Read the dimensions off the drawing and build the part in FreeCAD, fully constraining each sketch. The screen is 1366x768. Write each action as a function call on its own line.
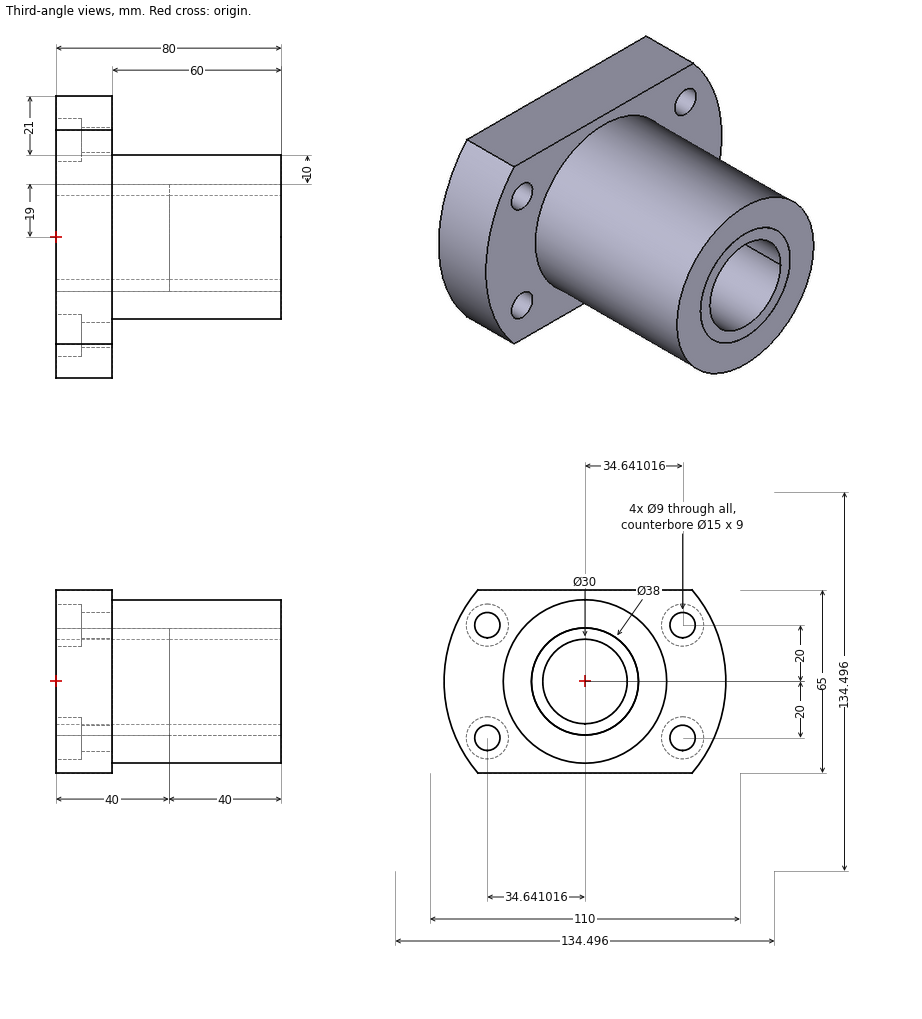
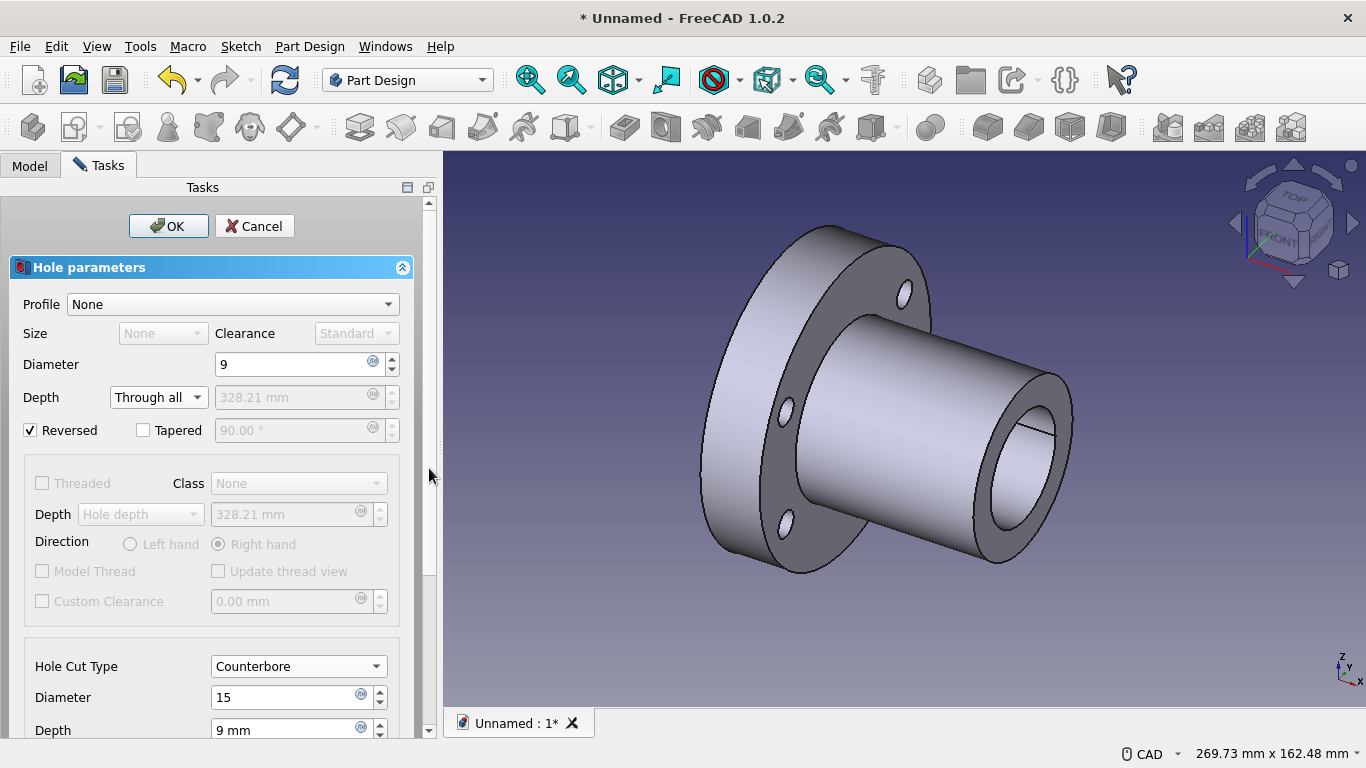
click(169, 226)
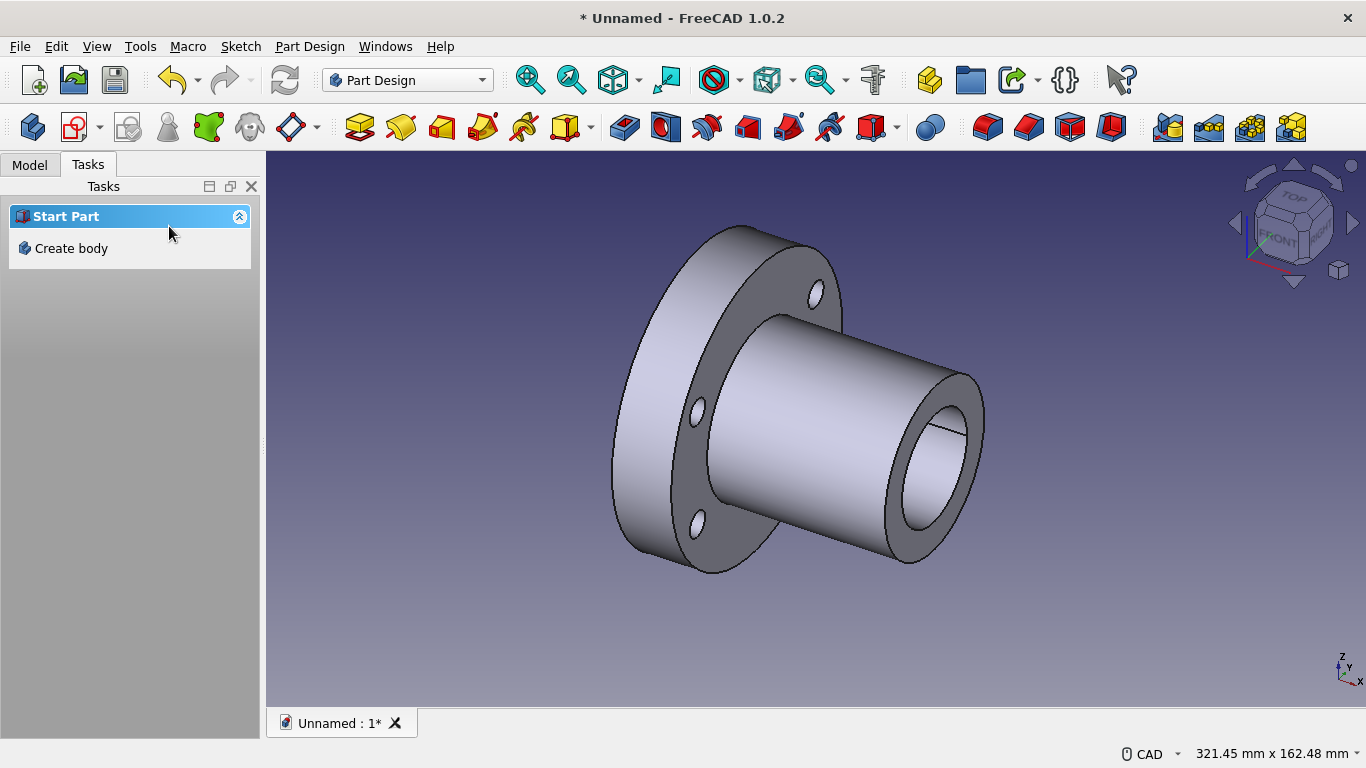
click(74, 128)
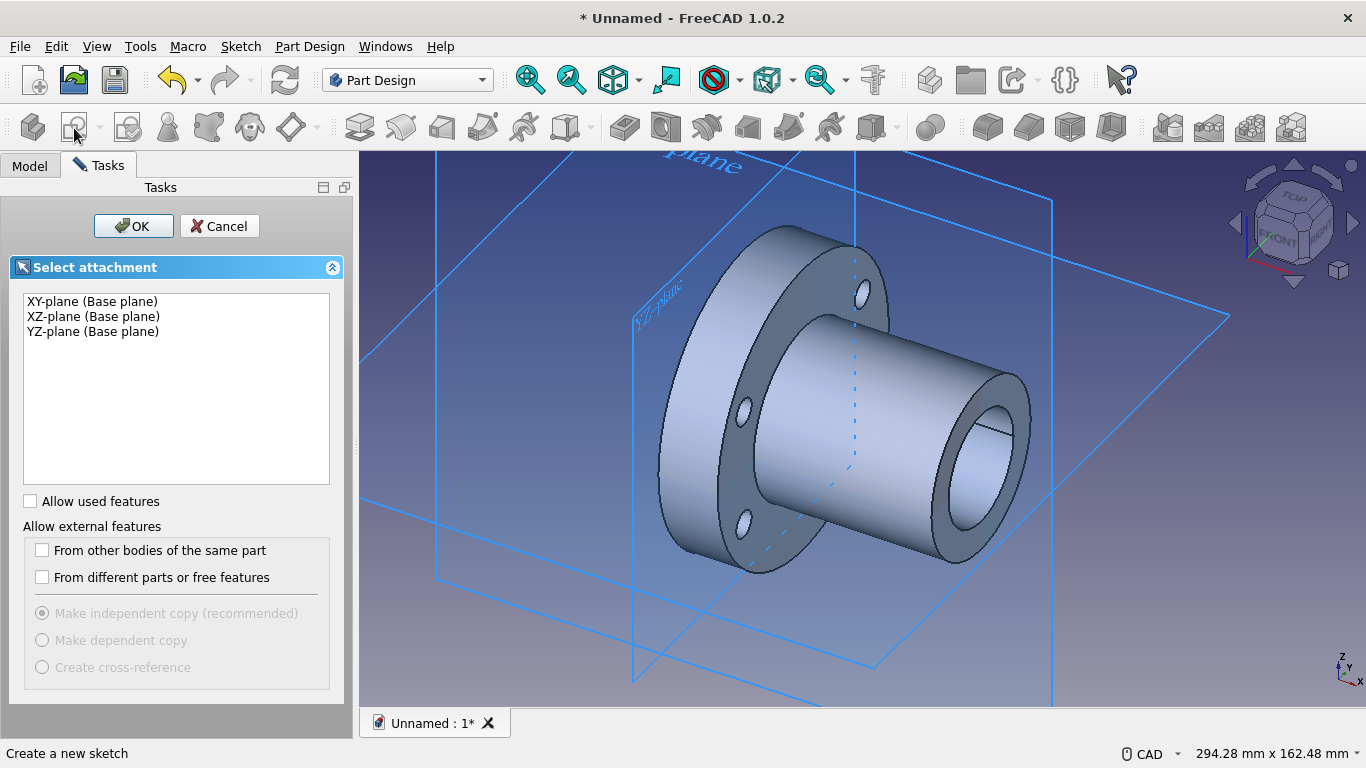
click(84, 332)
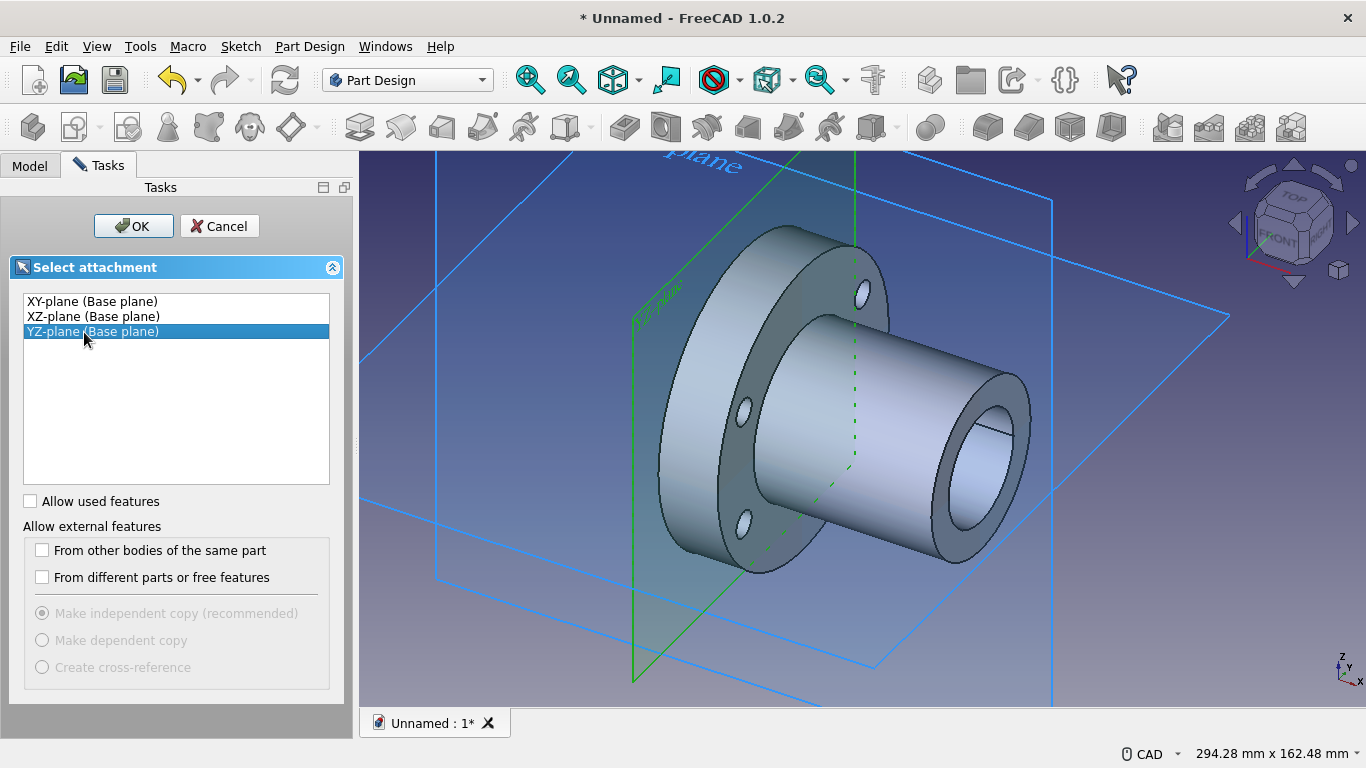
click(134, 226)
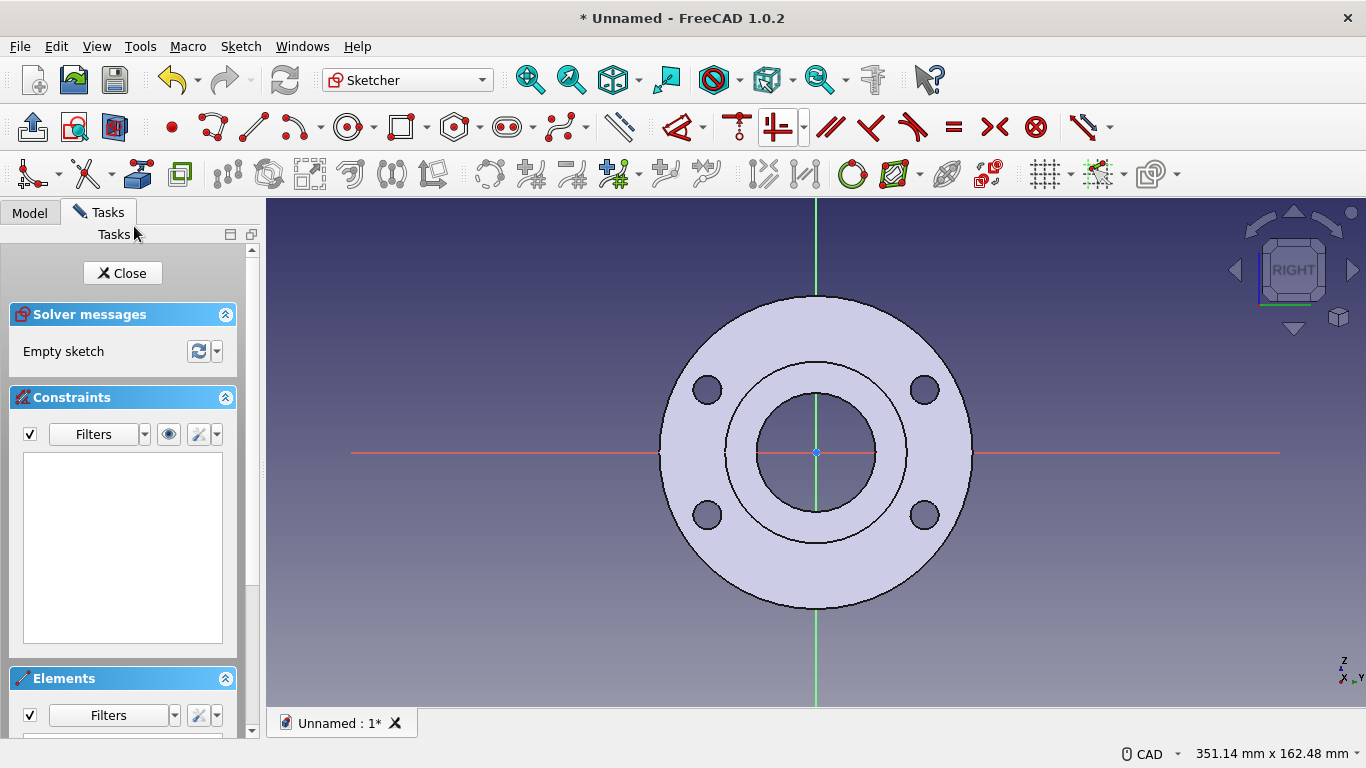
click(115, 128)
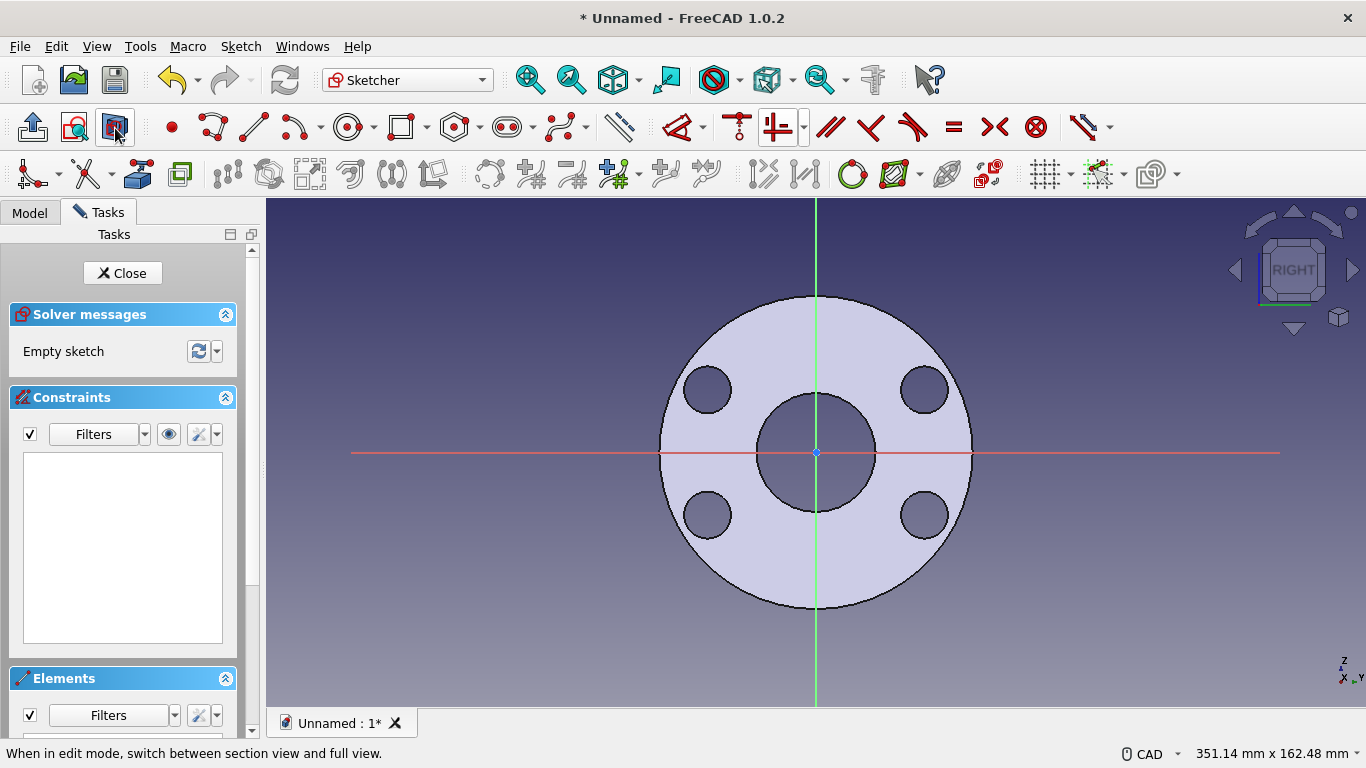
scroll(438, 452, down, 1)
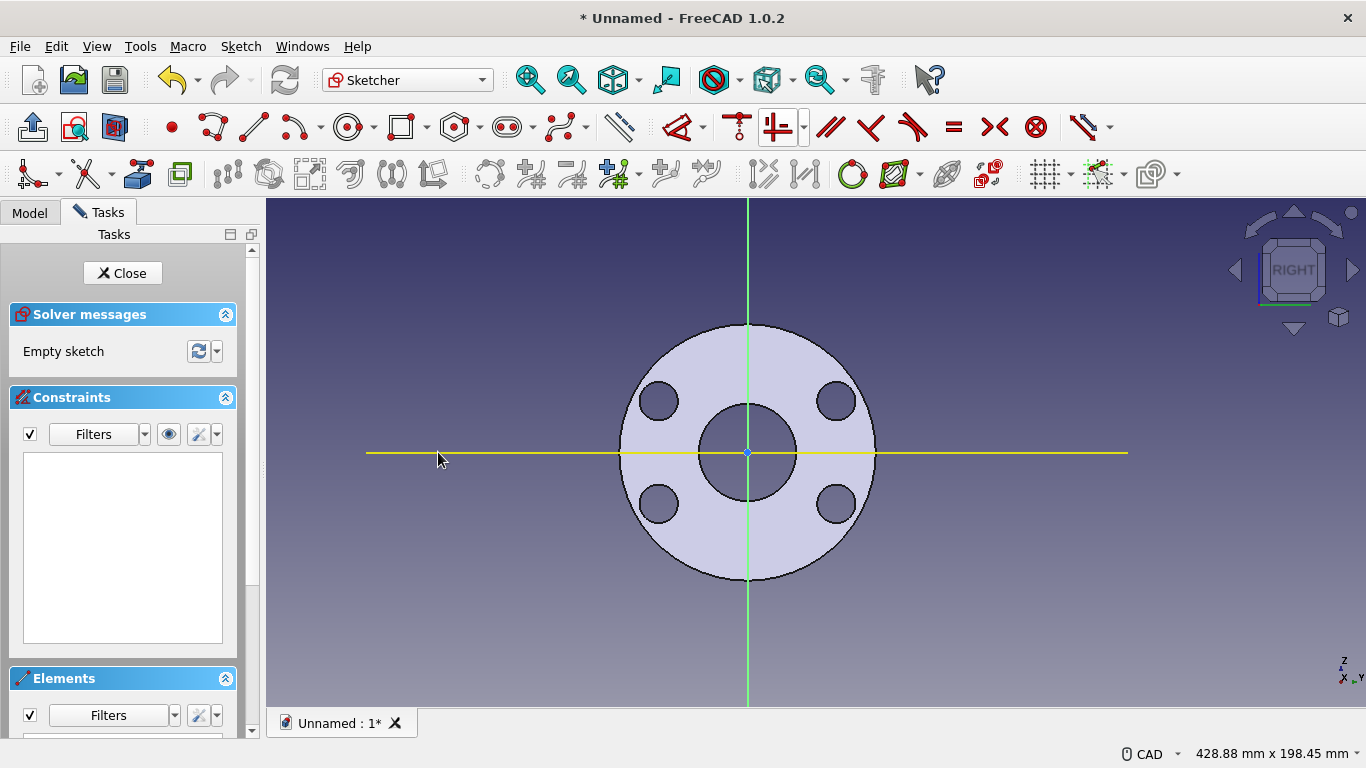
key(g)
key(v)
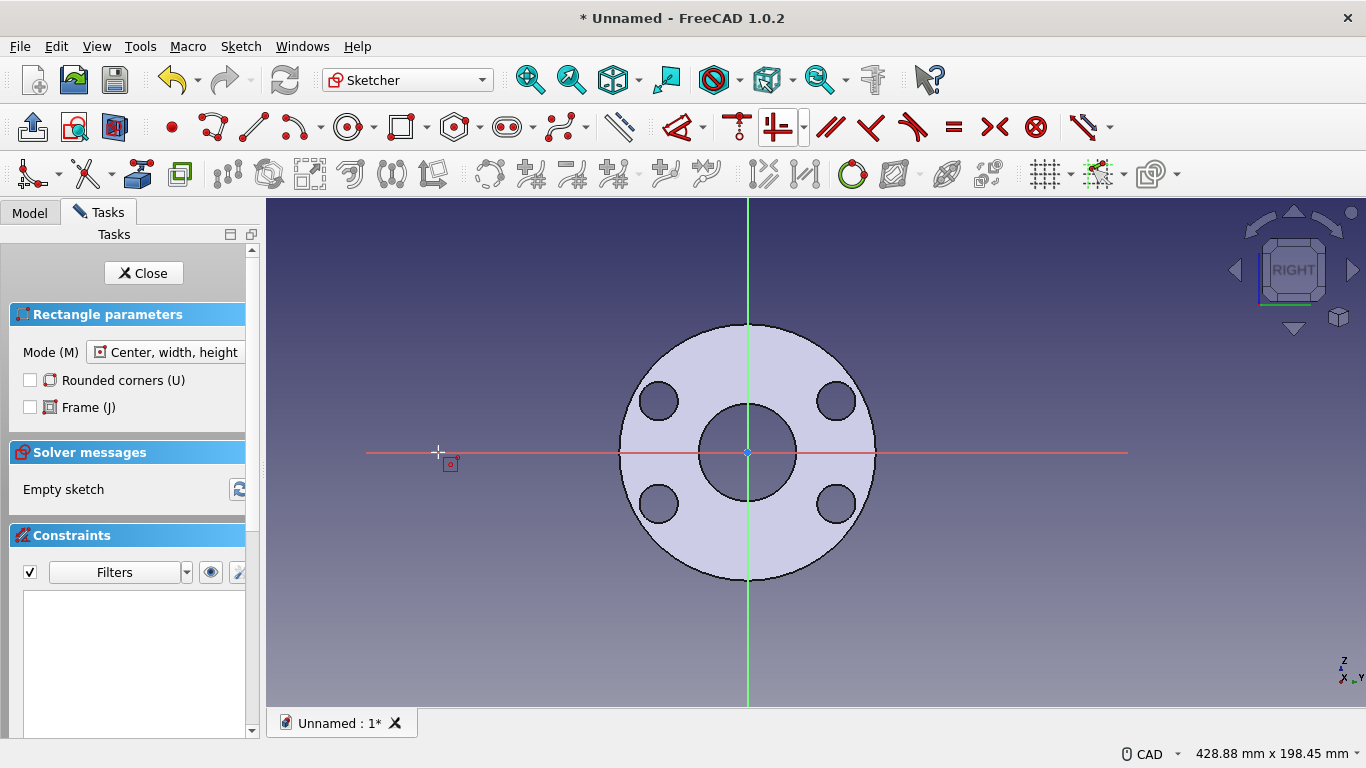
click(748, 452)
click(920, 280)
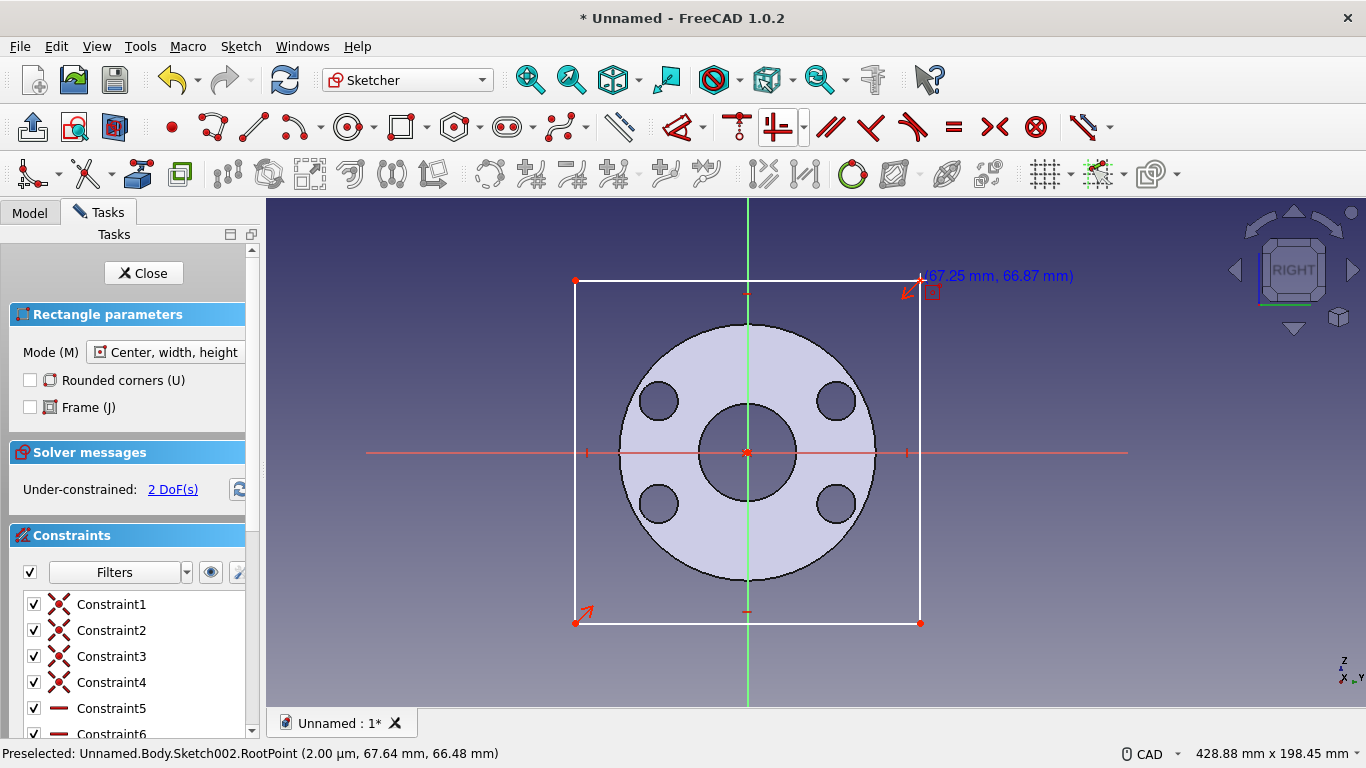
click(748, 452)
click(889, 369)
key(Escape)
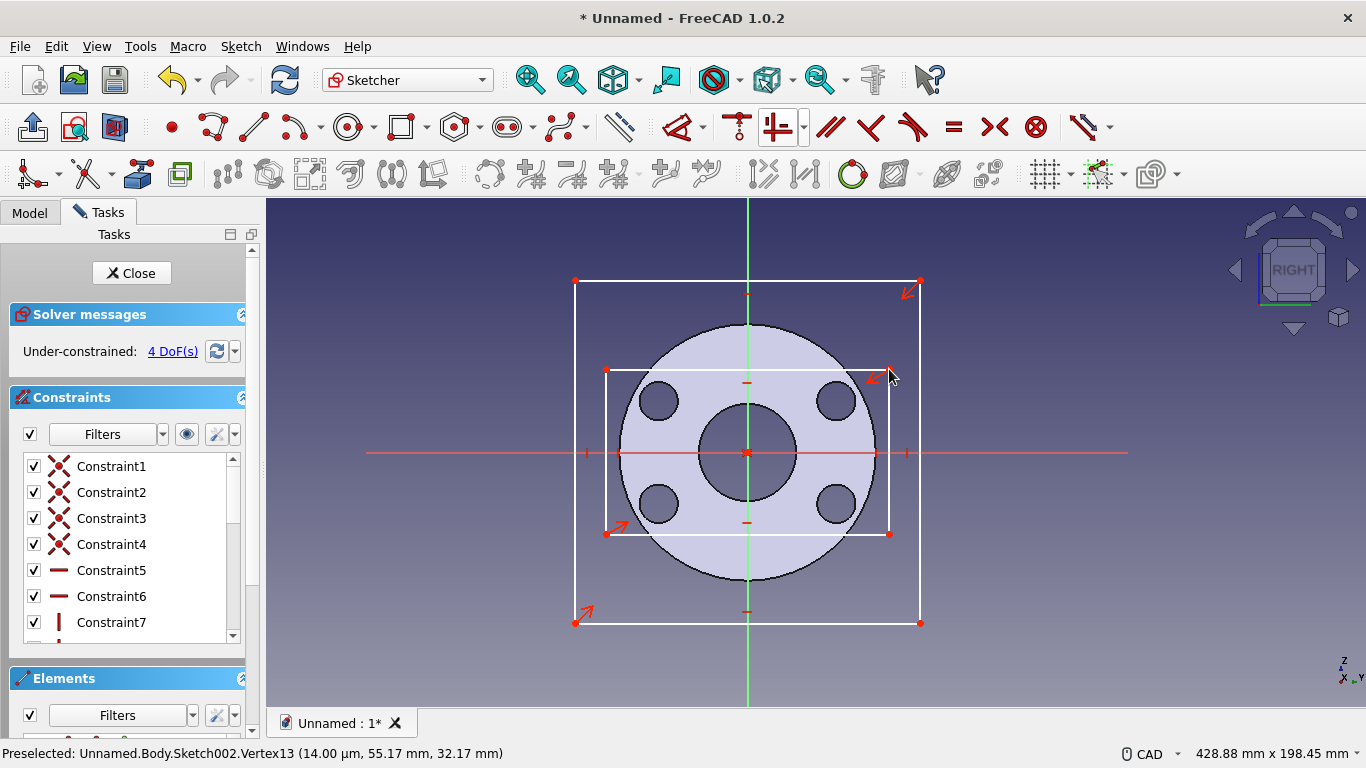
click(676, 128)